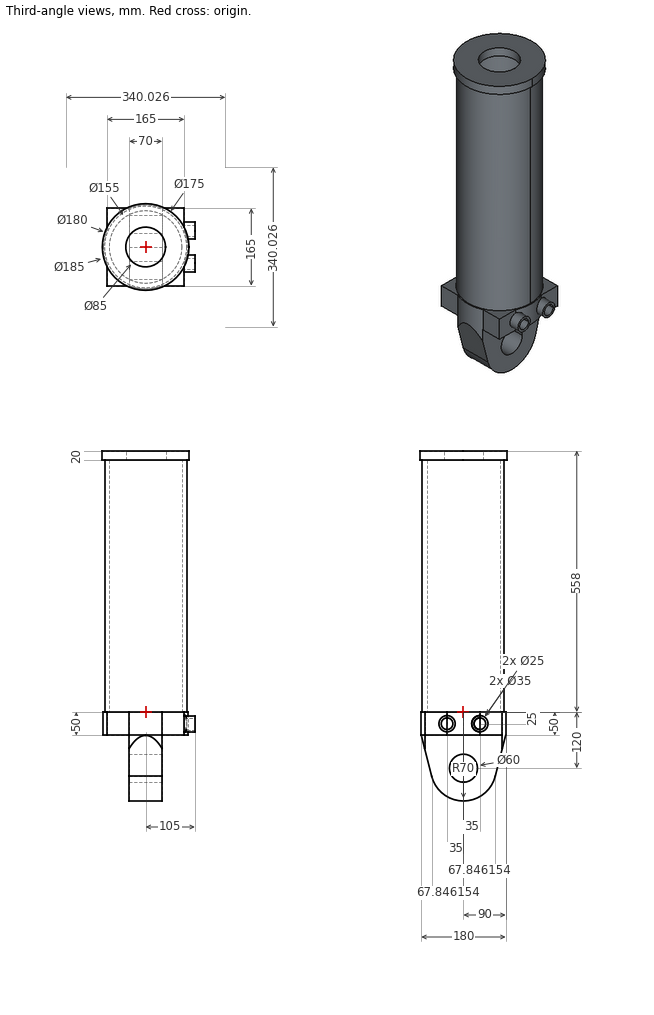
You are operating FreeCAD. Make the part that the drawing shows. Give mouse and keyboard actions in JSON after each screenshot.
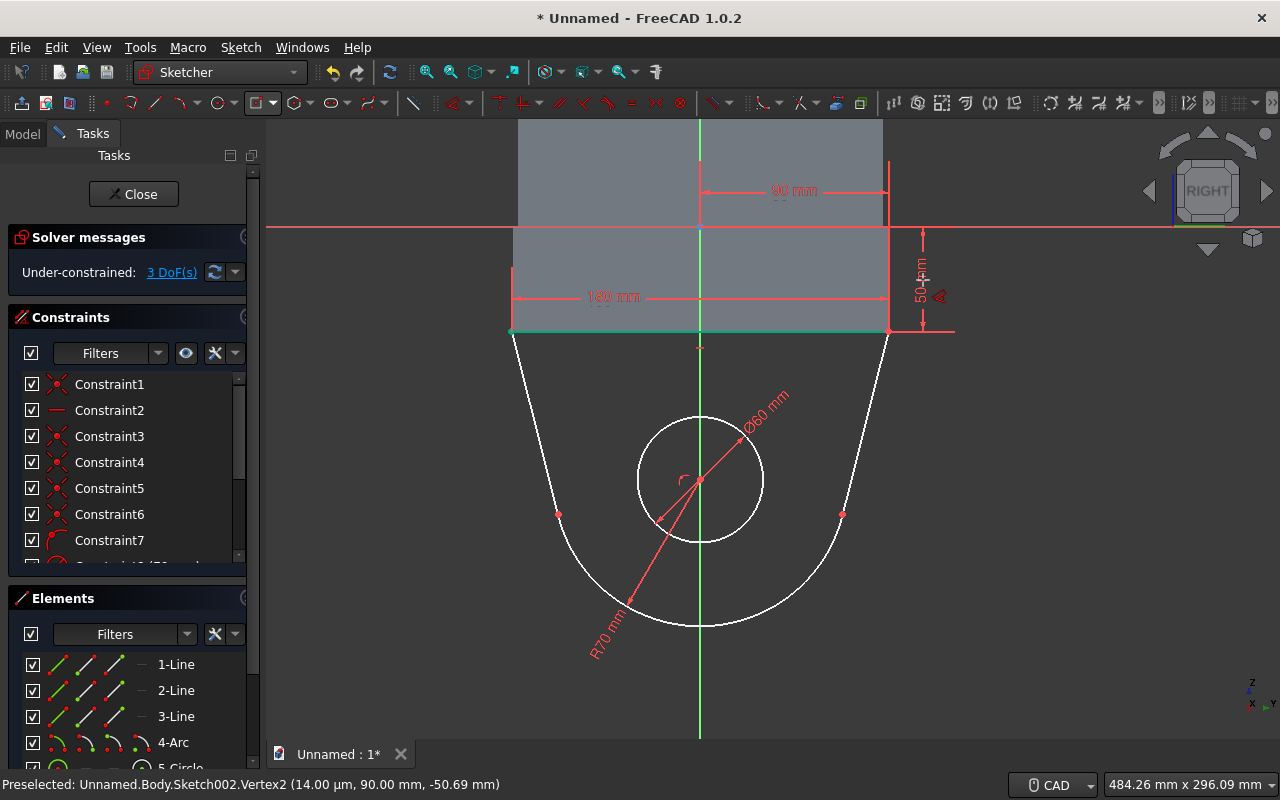
{"action": "left_click", "coordinate": [700, 480]}
{"action": "left_click", "coordinate": [734, 353]}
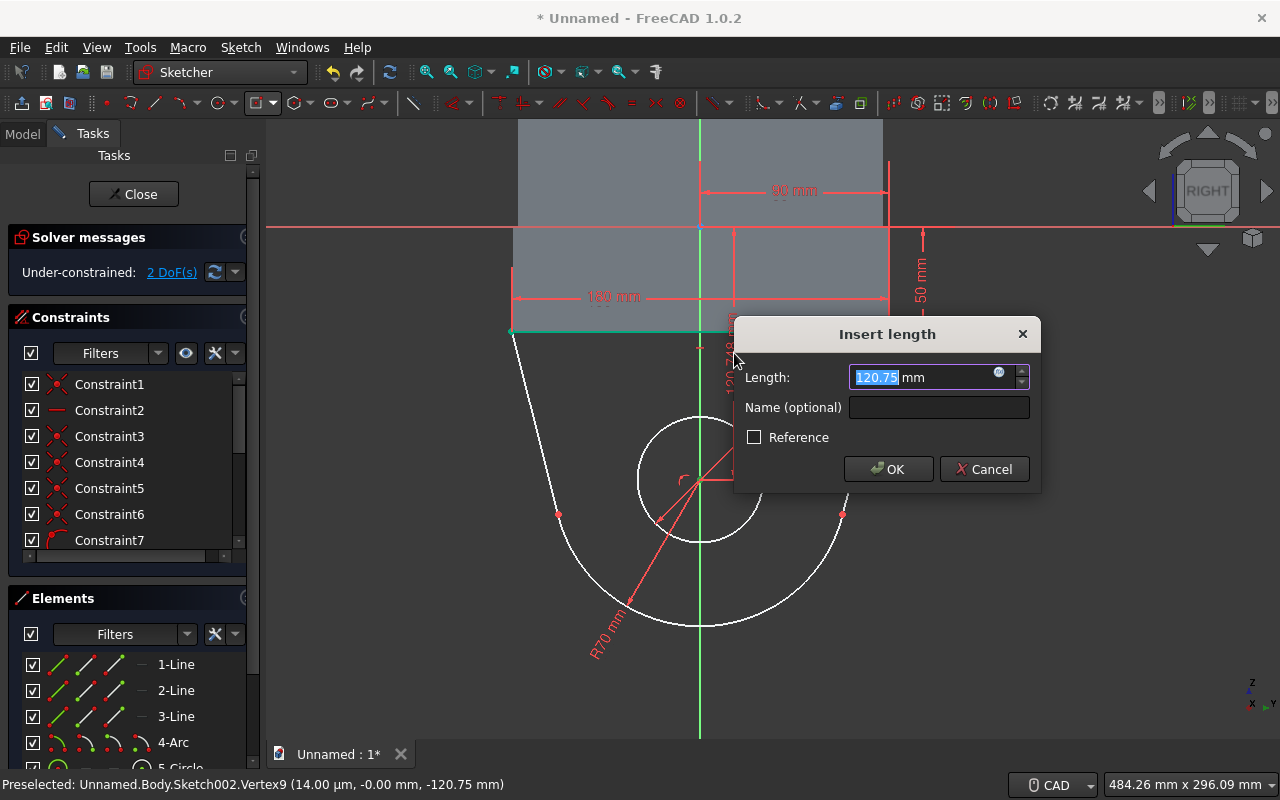
{"action": "type", "text": "120"}
{"action": "key", "text": "Return"}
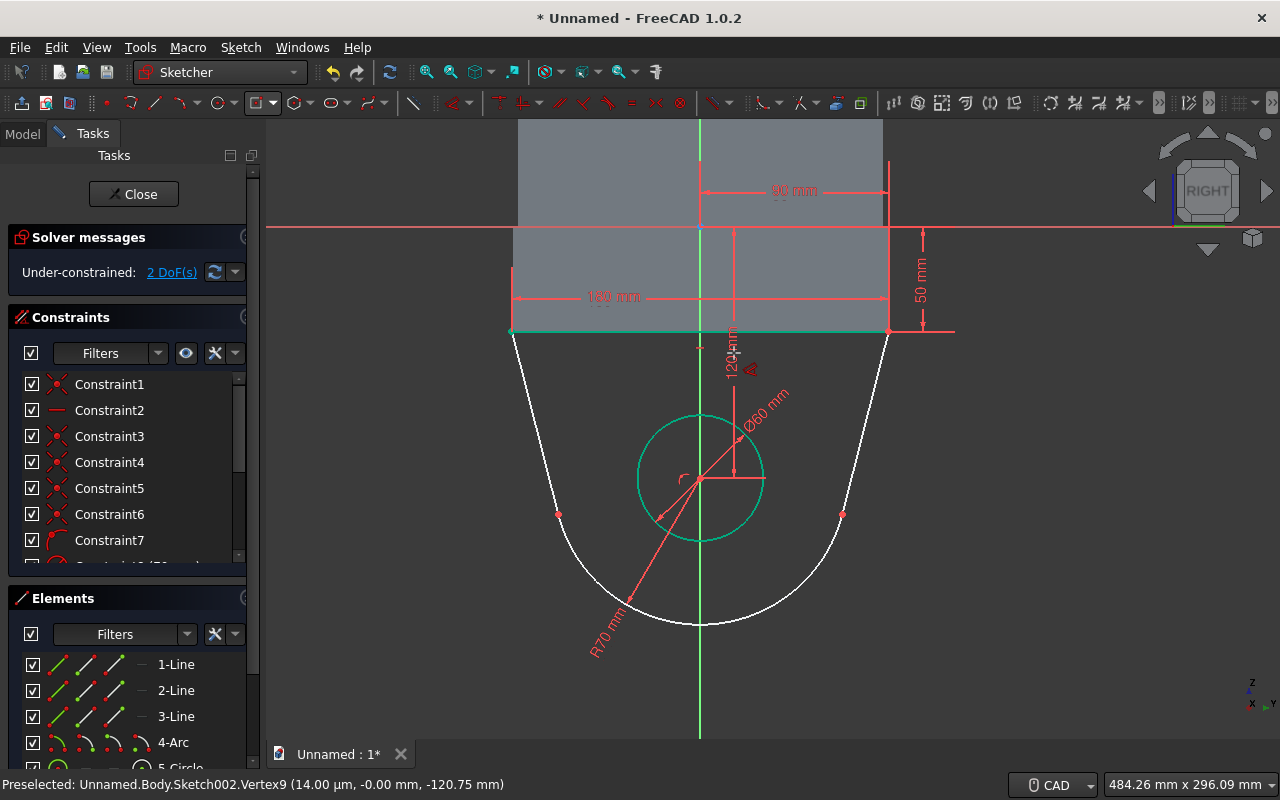
{"action": "left_click", "coordinate": [842, 515]}
{"action": "left_click", "coordinate": [722, 193]}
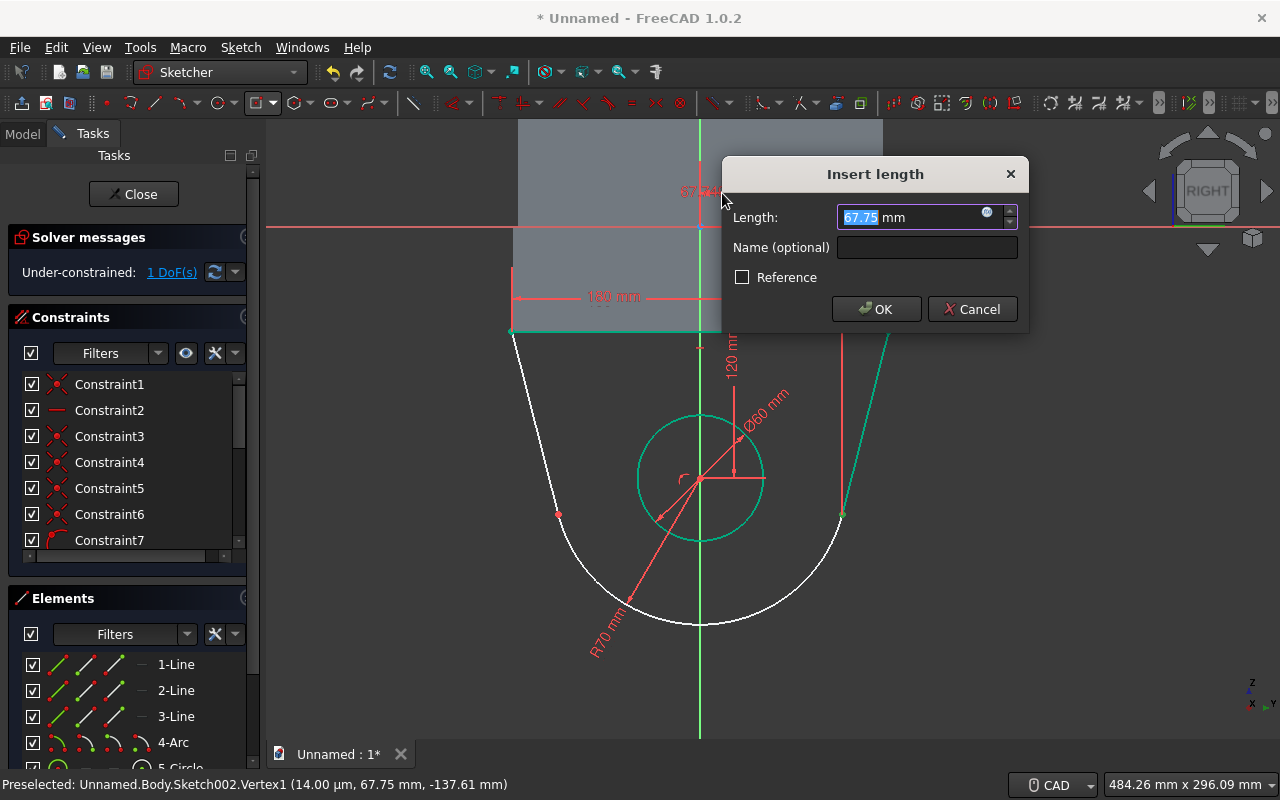
{"action": "type", "text": "67.846154"}
{"action": "key", "text": "Return"}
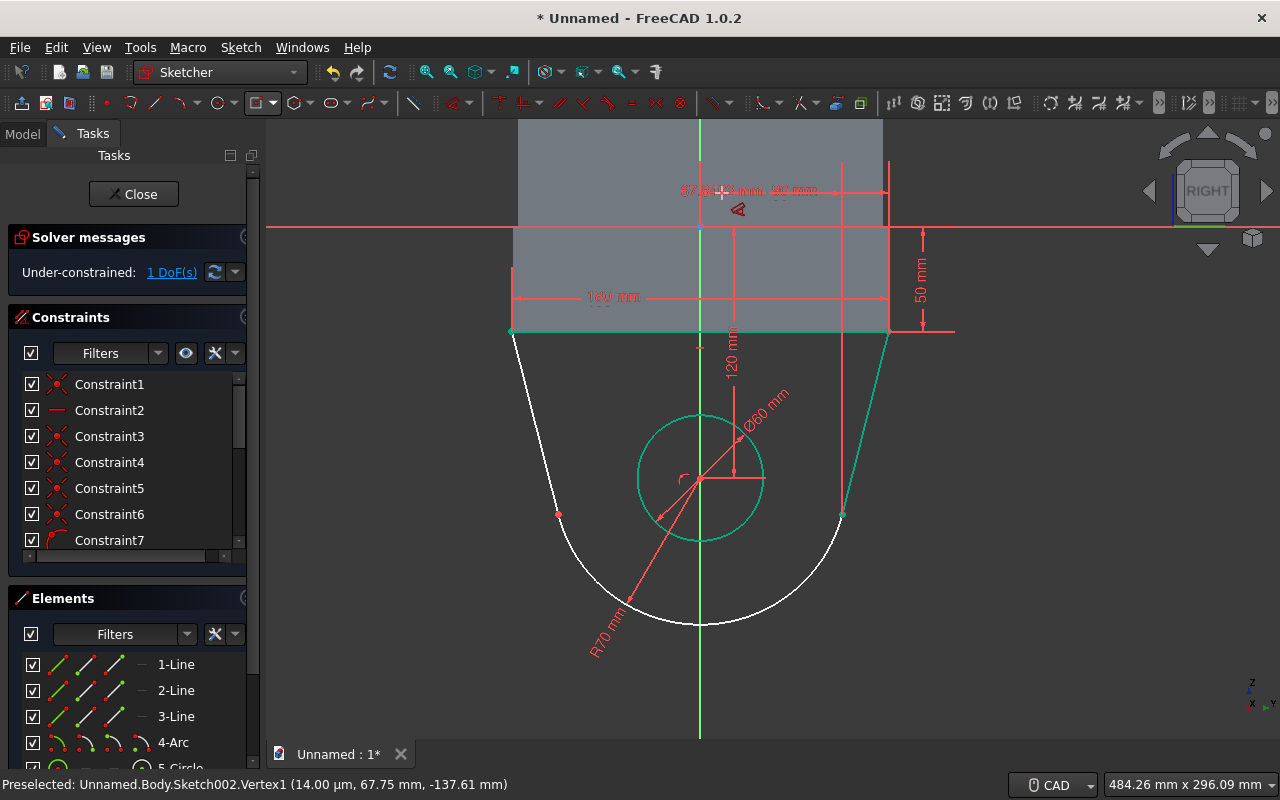
{"action": "left_click", "coordinate": [558, 515]}
{"action": "left_click", "coordinate": [629, 193]}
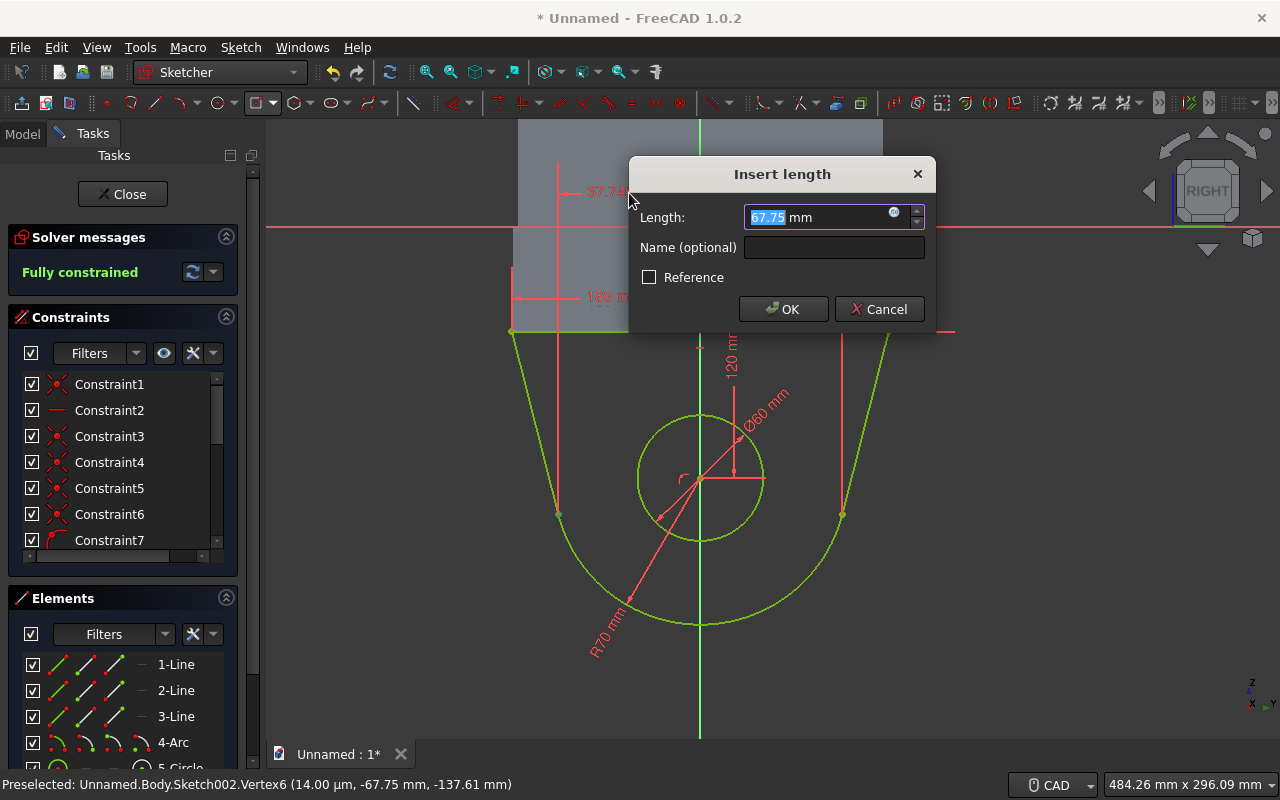
{"action": "type", "text": "67.846154"}
{"action": "key", "text": "Return"}
{"action": "key", "text": "Escape"}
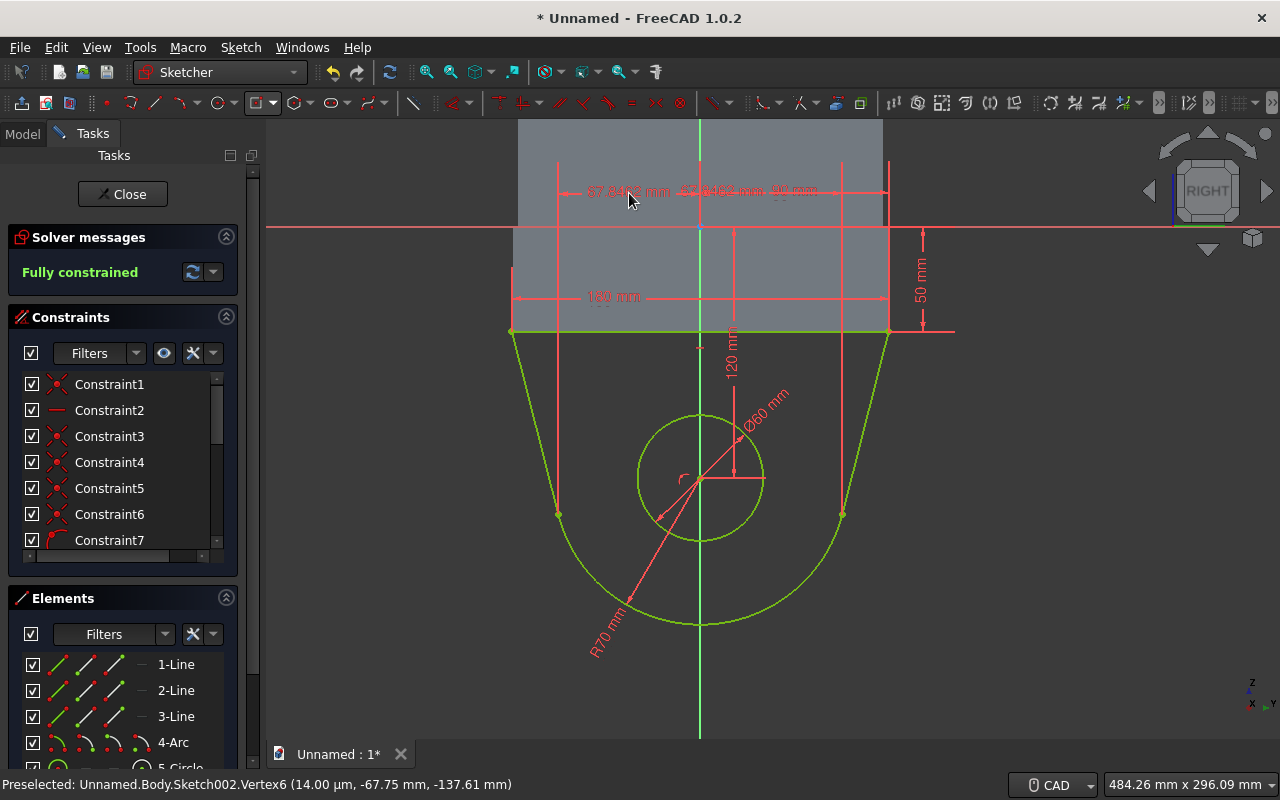
{"action": "left_click", "coordinate": [123, 194]}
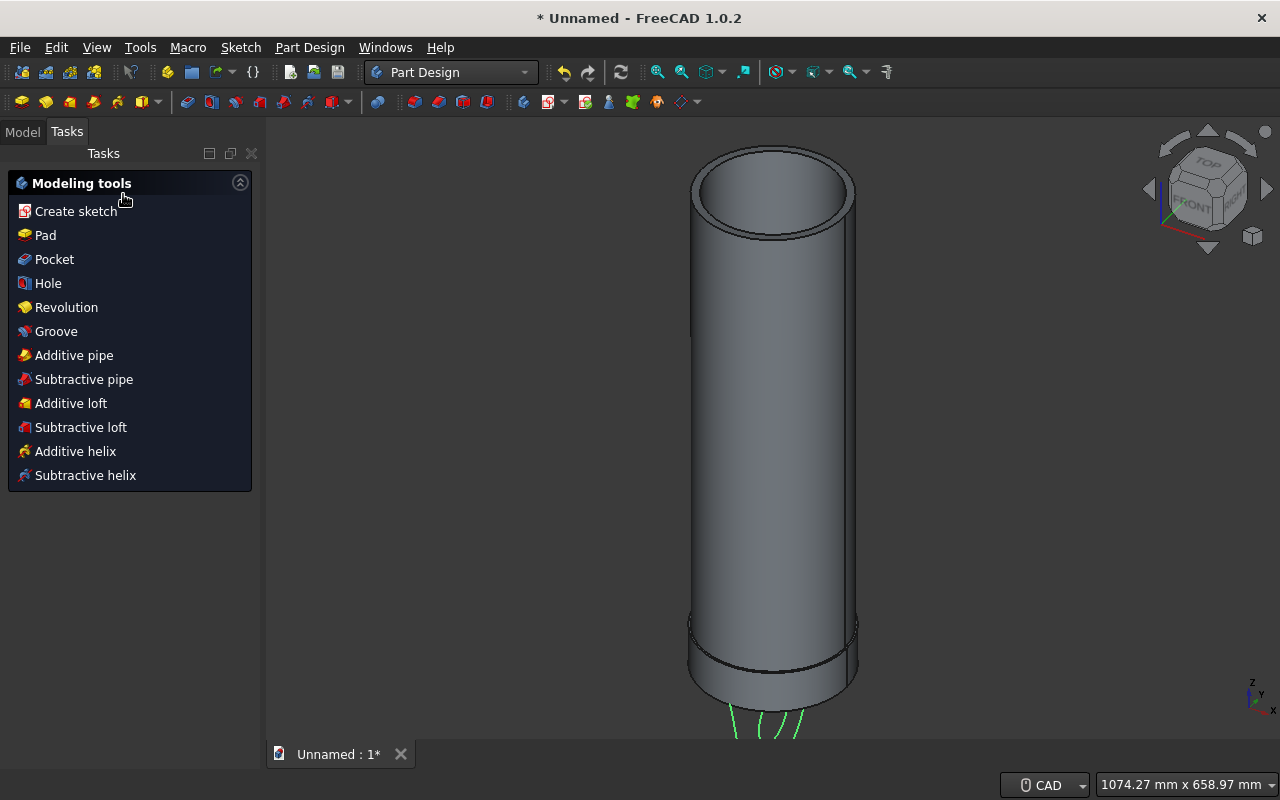
{"action": "left_click", "coordinate": [22, 102]}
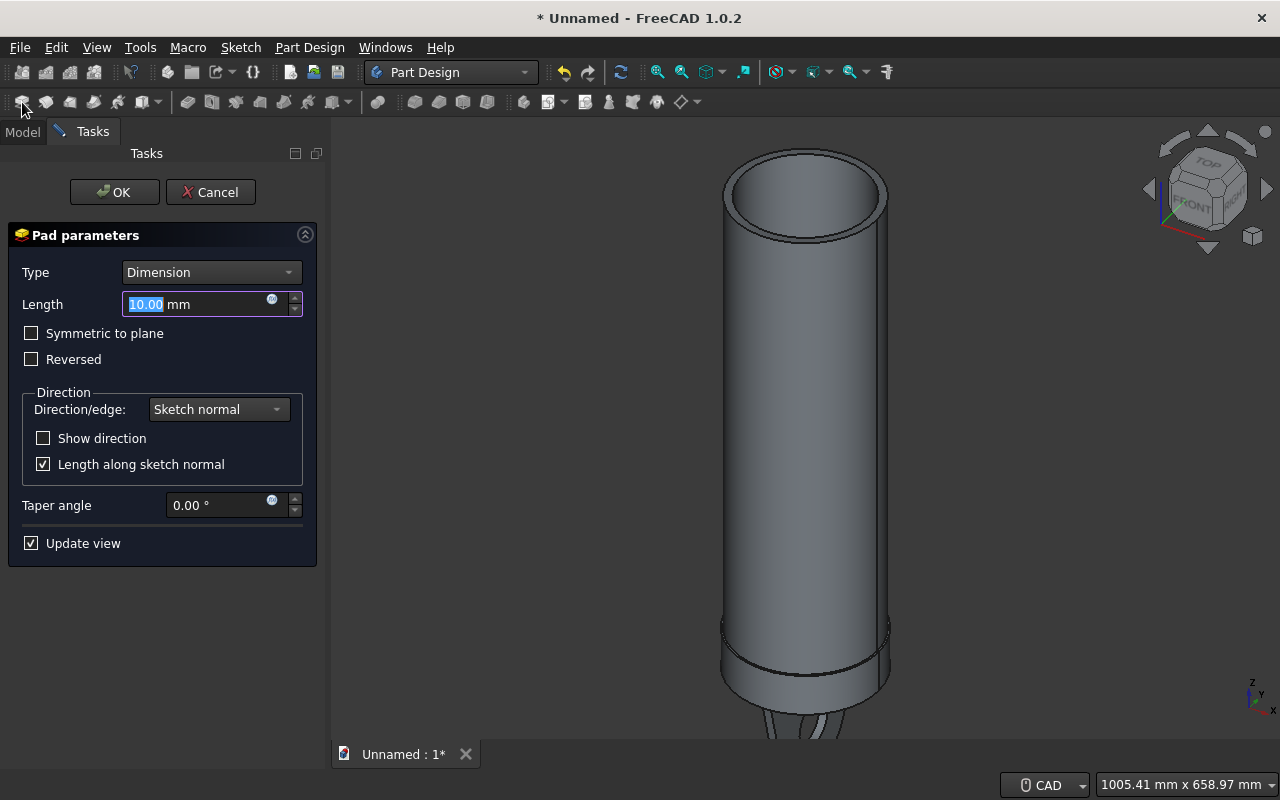
{"action": "type", "text": "70"}
{"action": "key", "text": "Tab"}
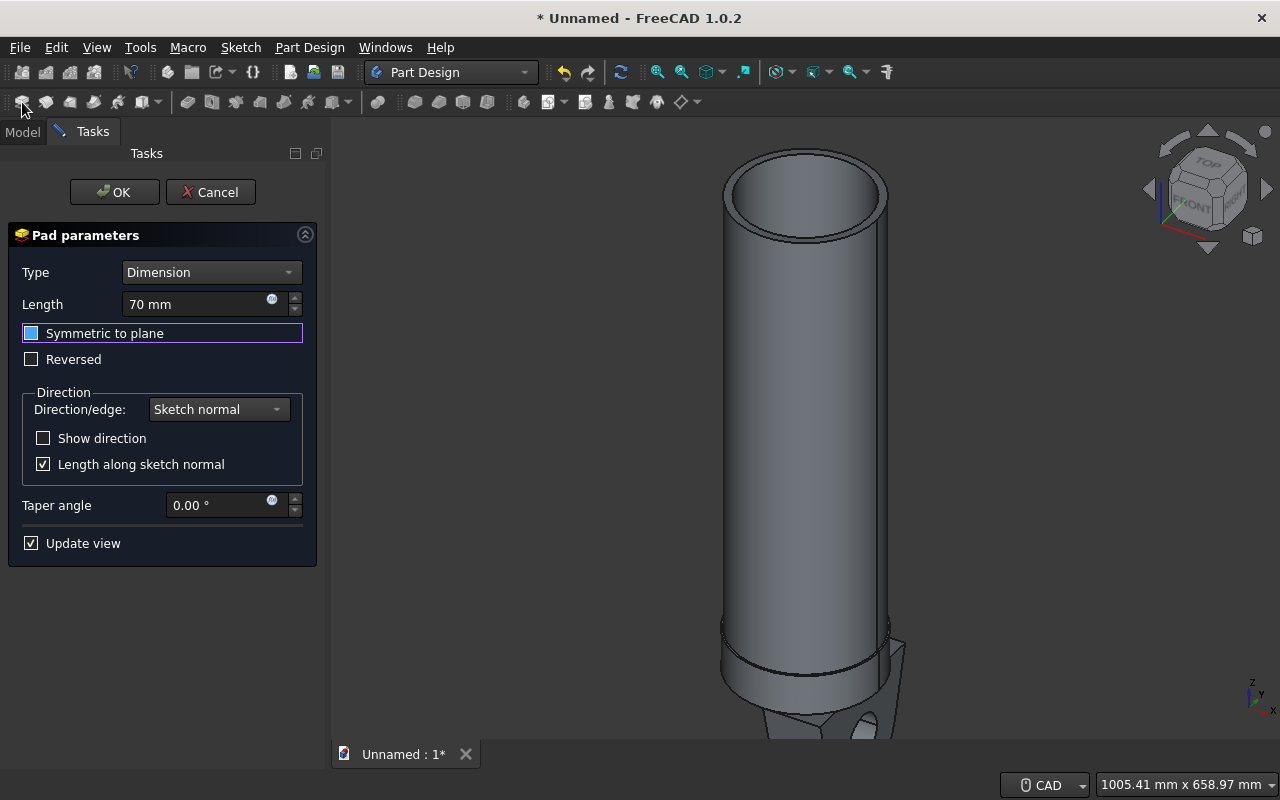
{"action": "left_click", "coordinate": [30, 333]}